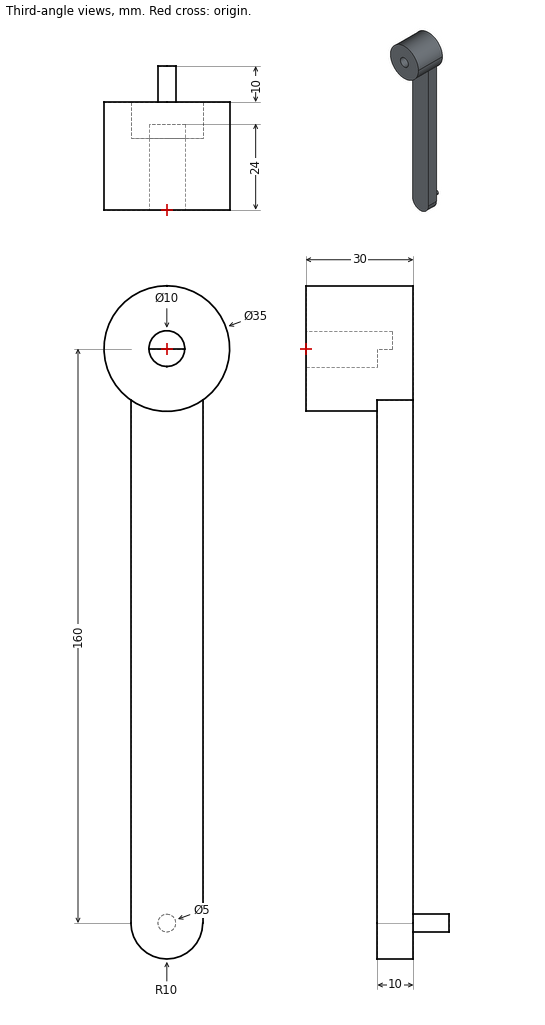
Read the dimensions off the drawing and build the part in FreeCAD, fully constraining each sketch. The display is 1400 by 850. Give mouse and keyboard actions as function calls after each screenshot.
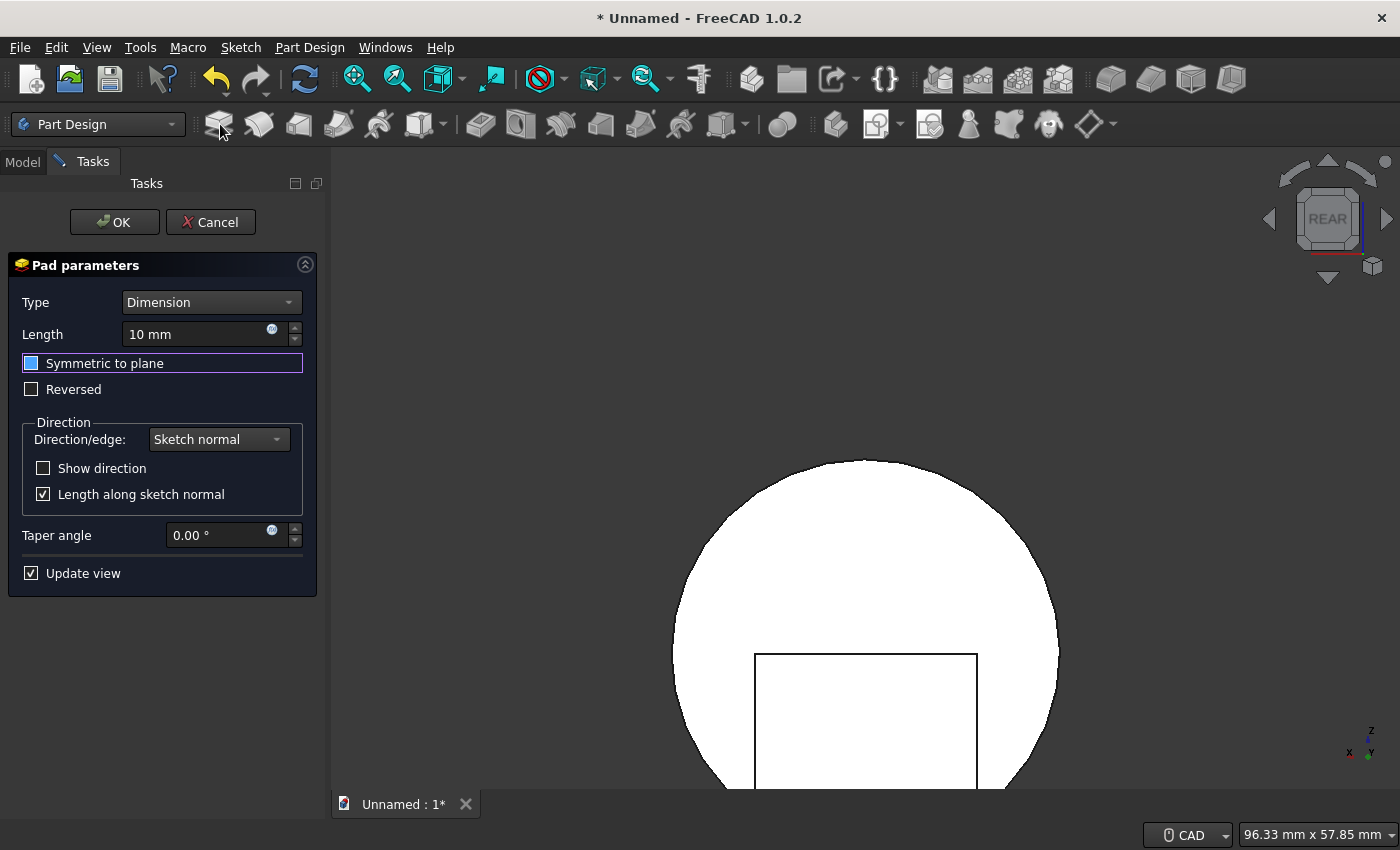
click(30, 389)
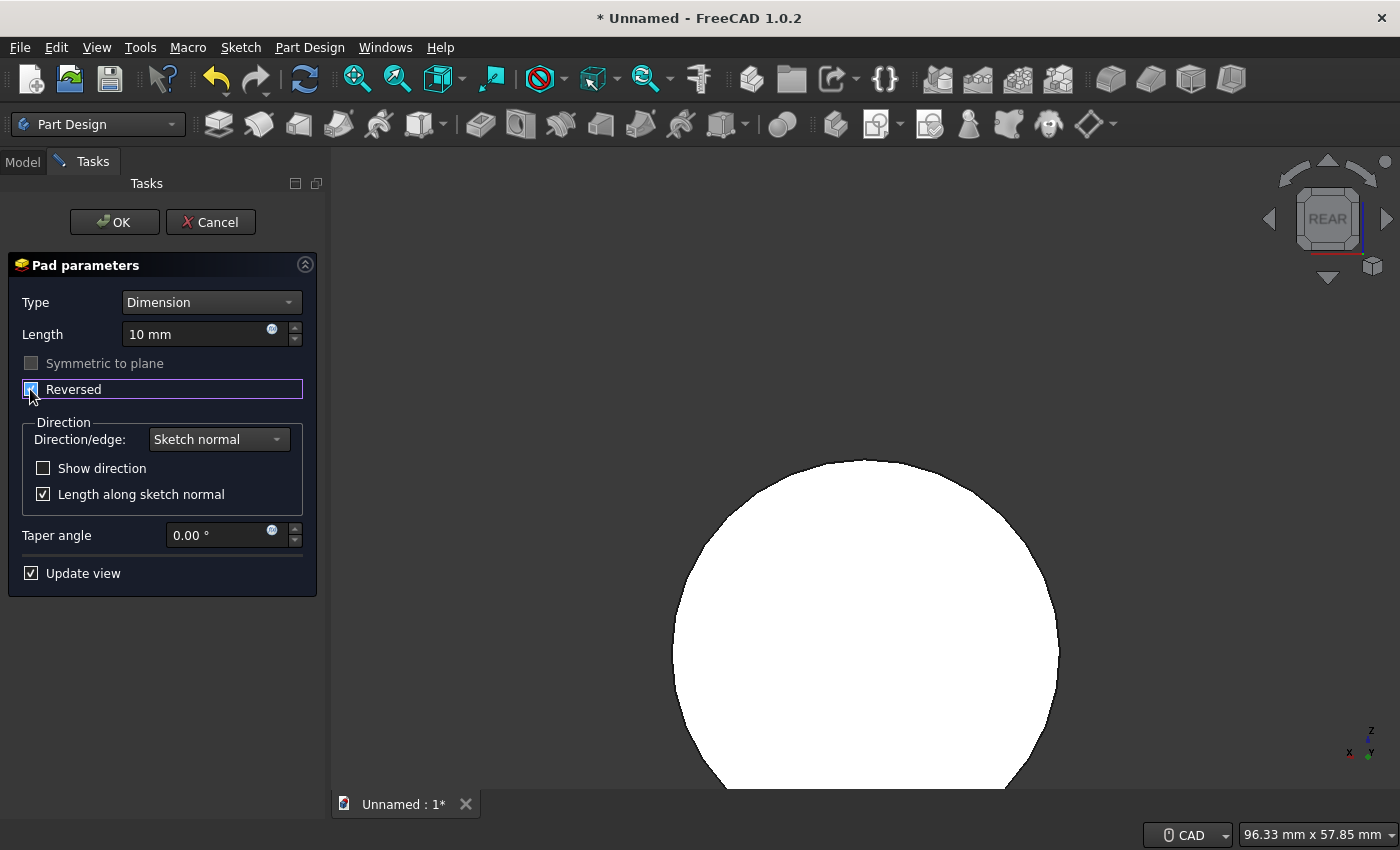
click(115, 222)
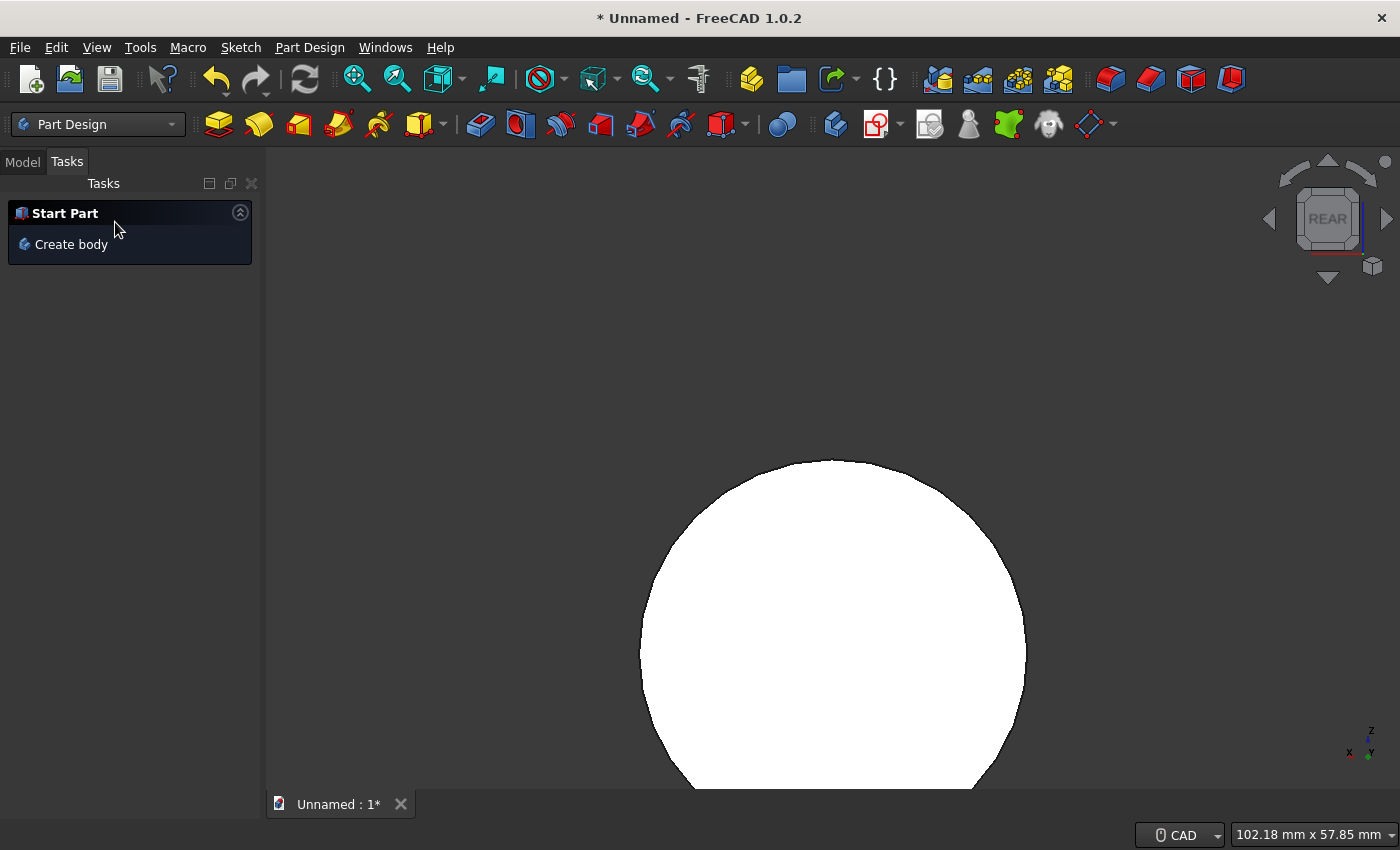
key(v)
key(f)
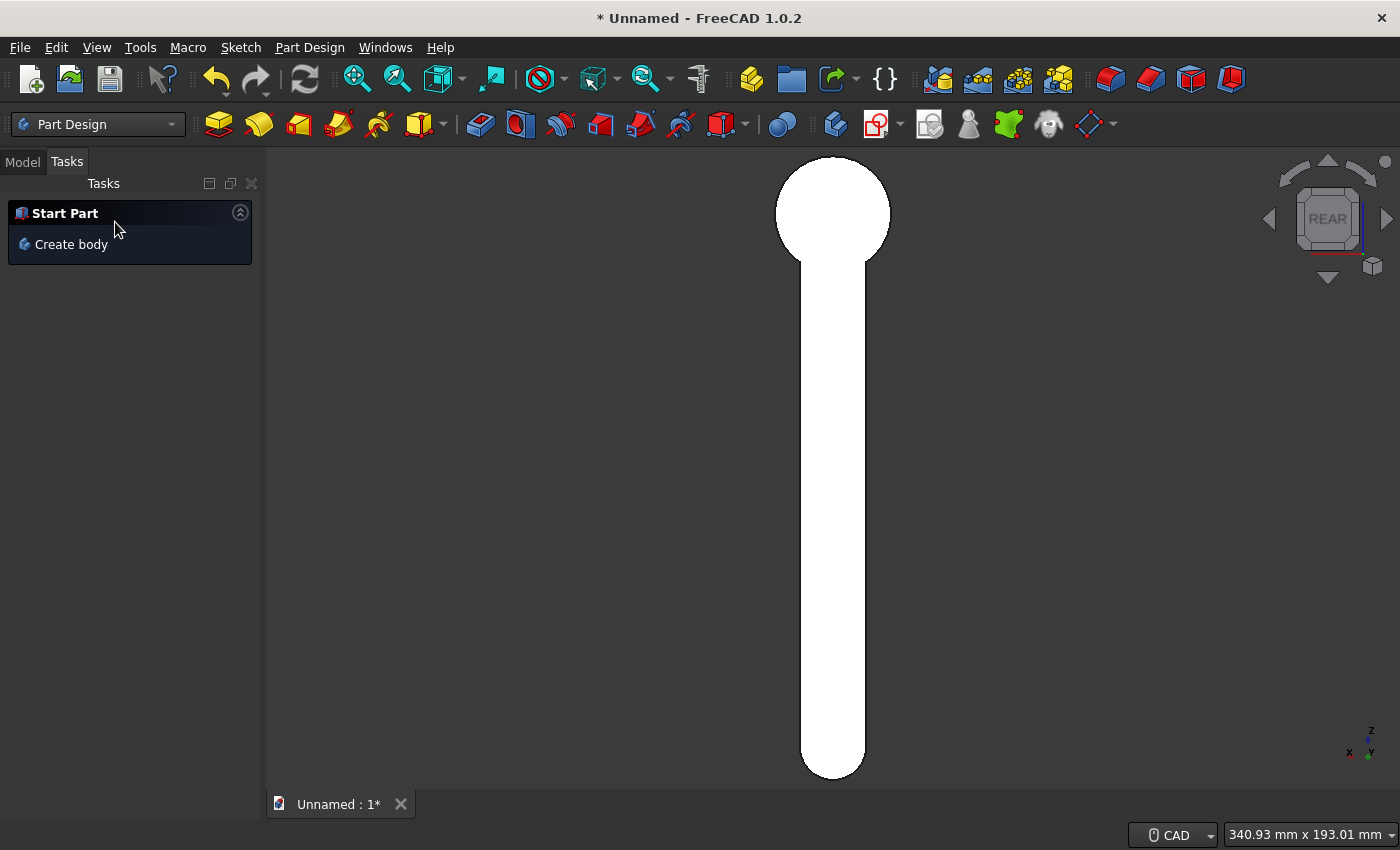
click(833, 200)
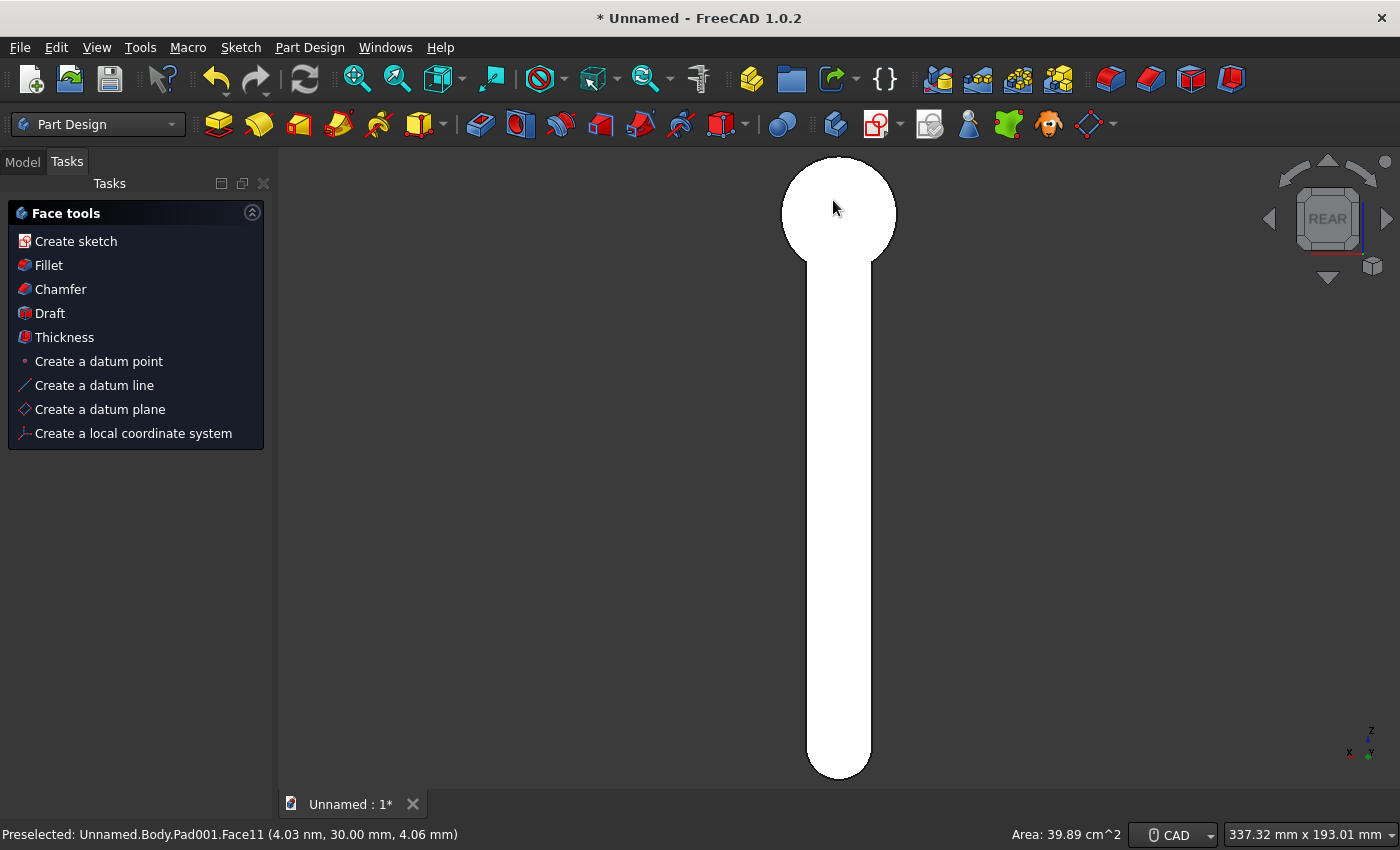
click(876, 124)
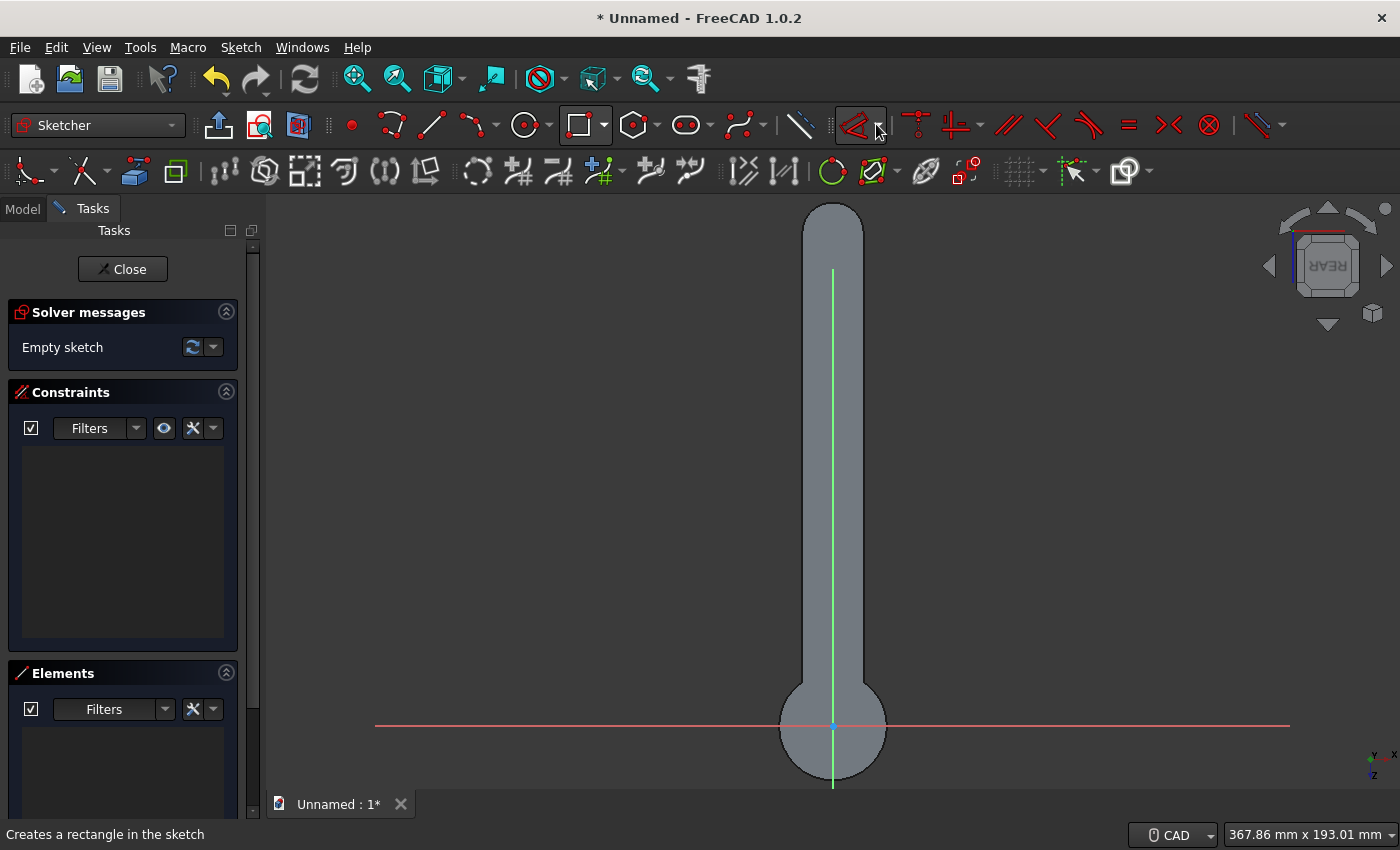
scroll(837, 222, up, 15)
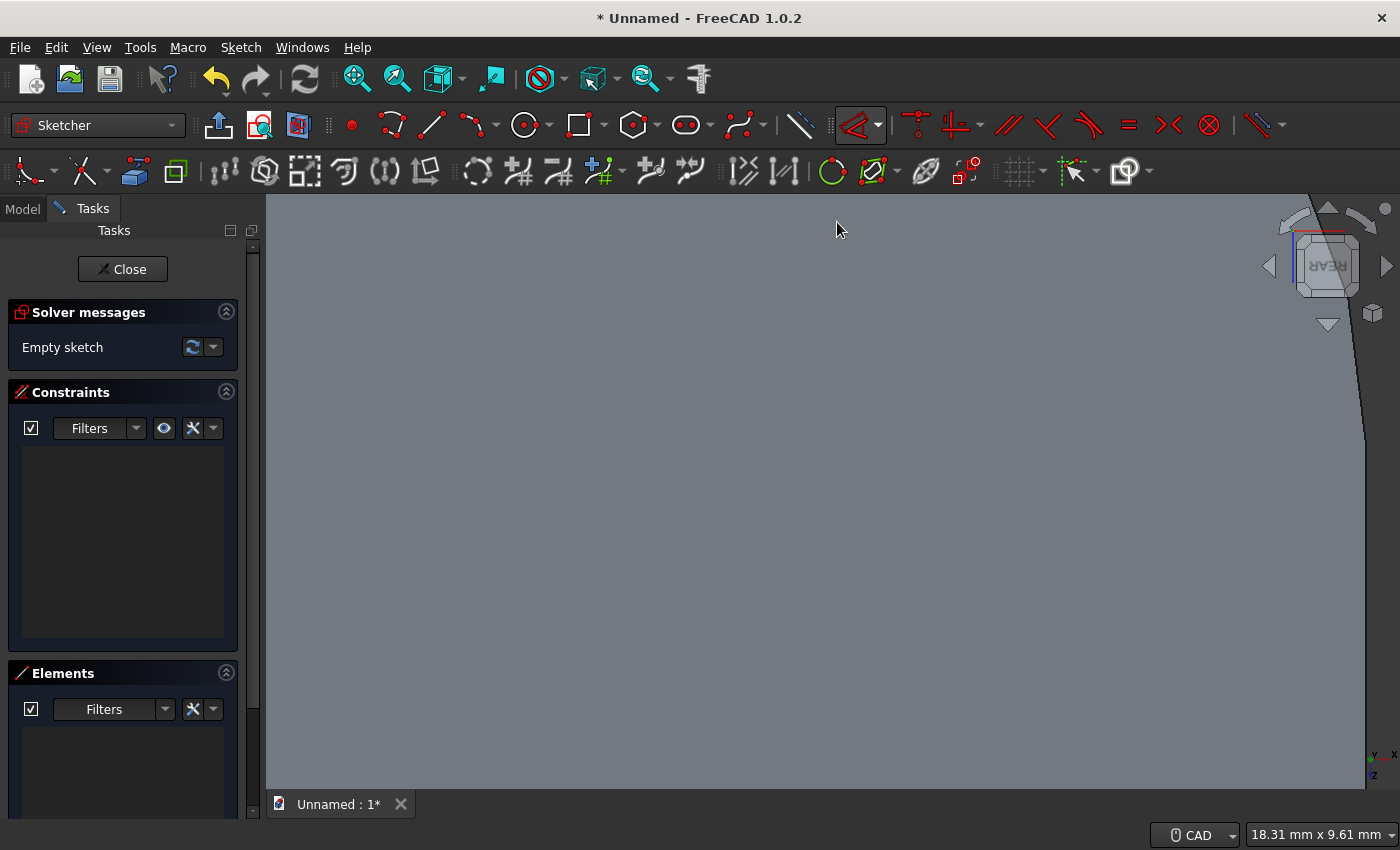
key(g)
key(c)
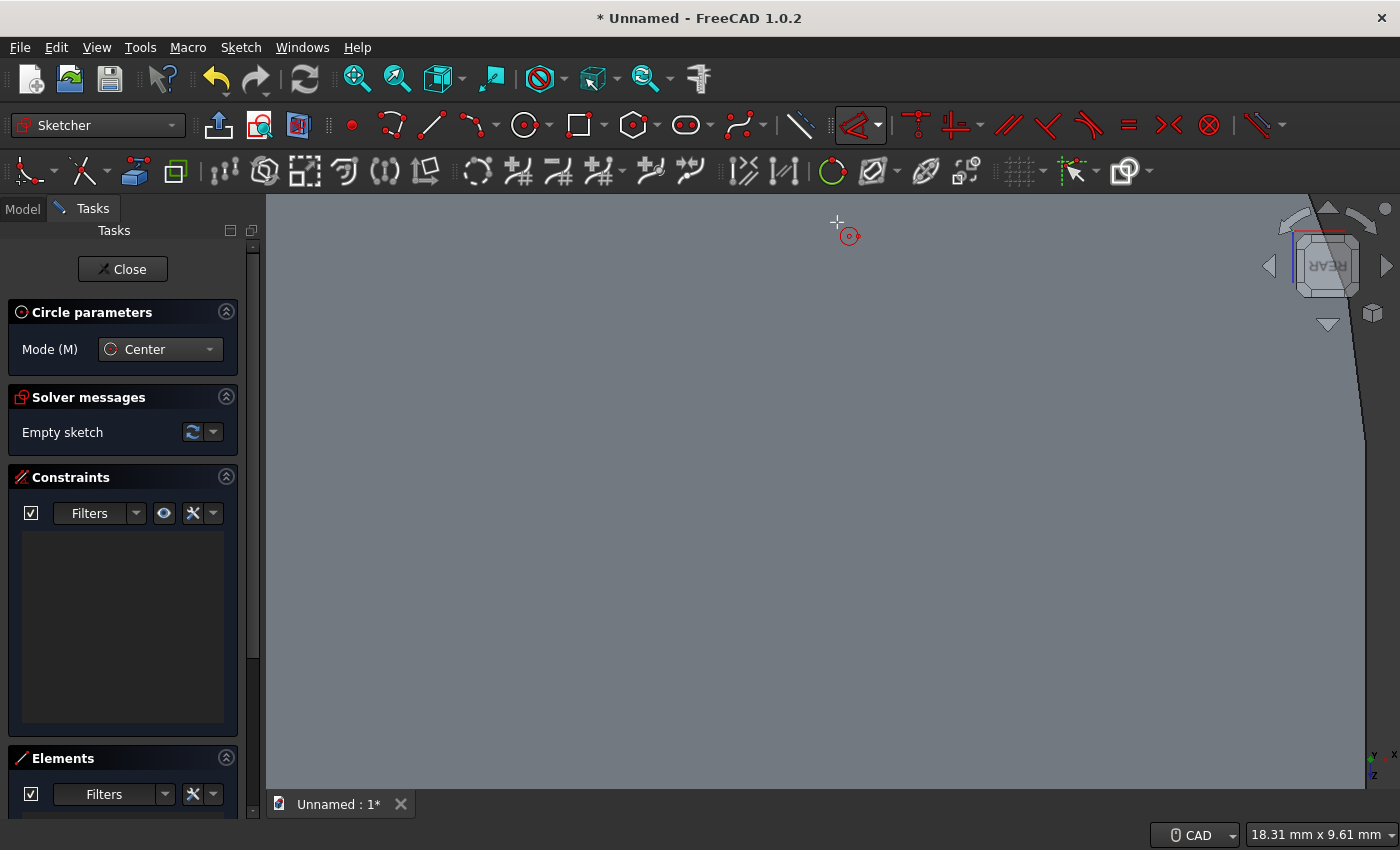
click(747, 446)
move(856, 337)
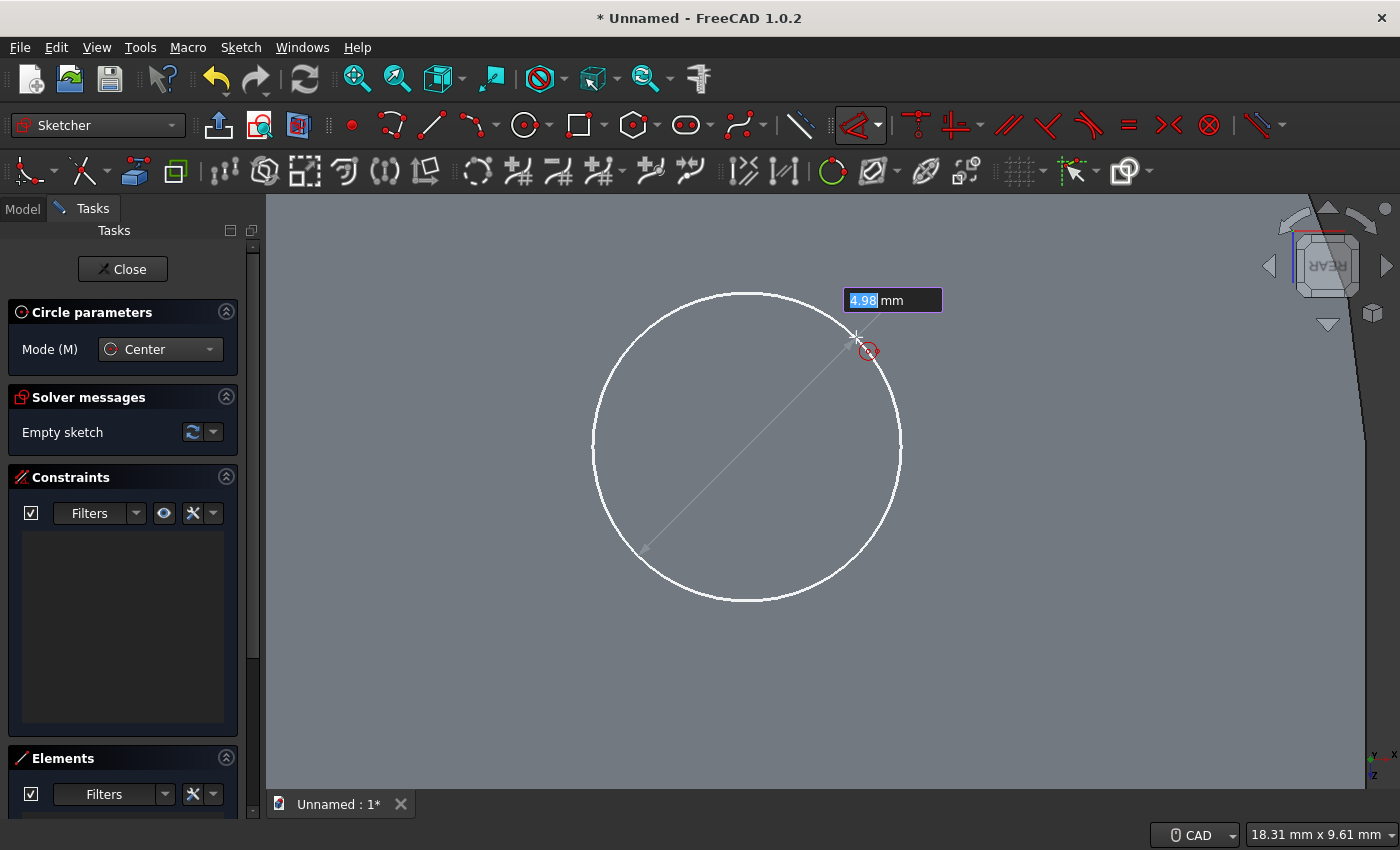
text(5)
key(Return)
key(Escape)